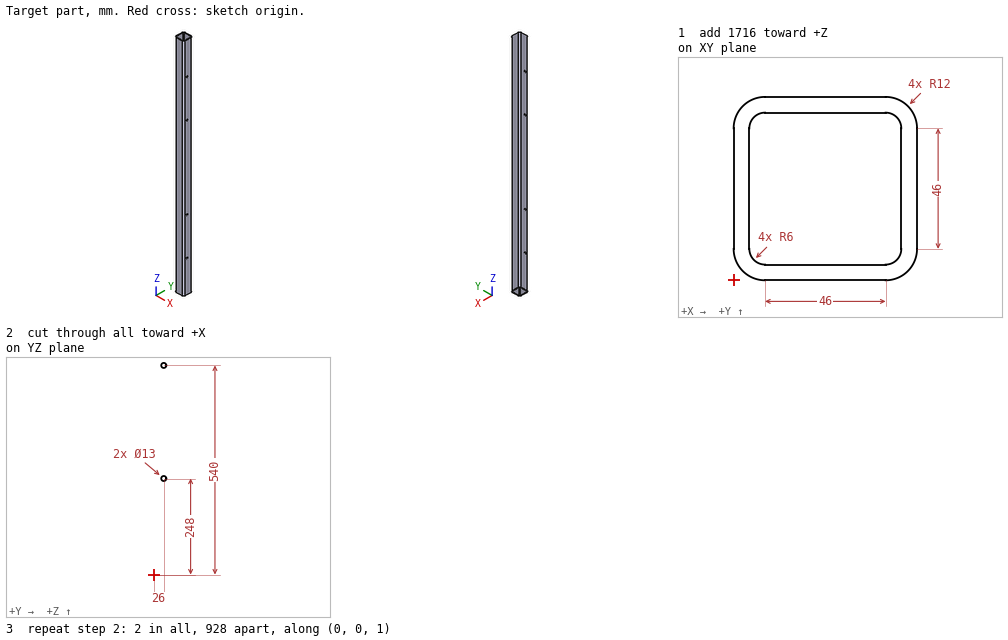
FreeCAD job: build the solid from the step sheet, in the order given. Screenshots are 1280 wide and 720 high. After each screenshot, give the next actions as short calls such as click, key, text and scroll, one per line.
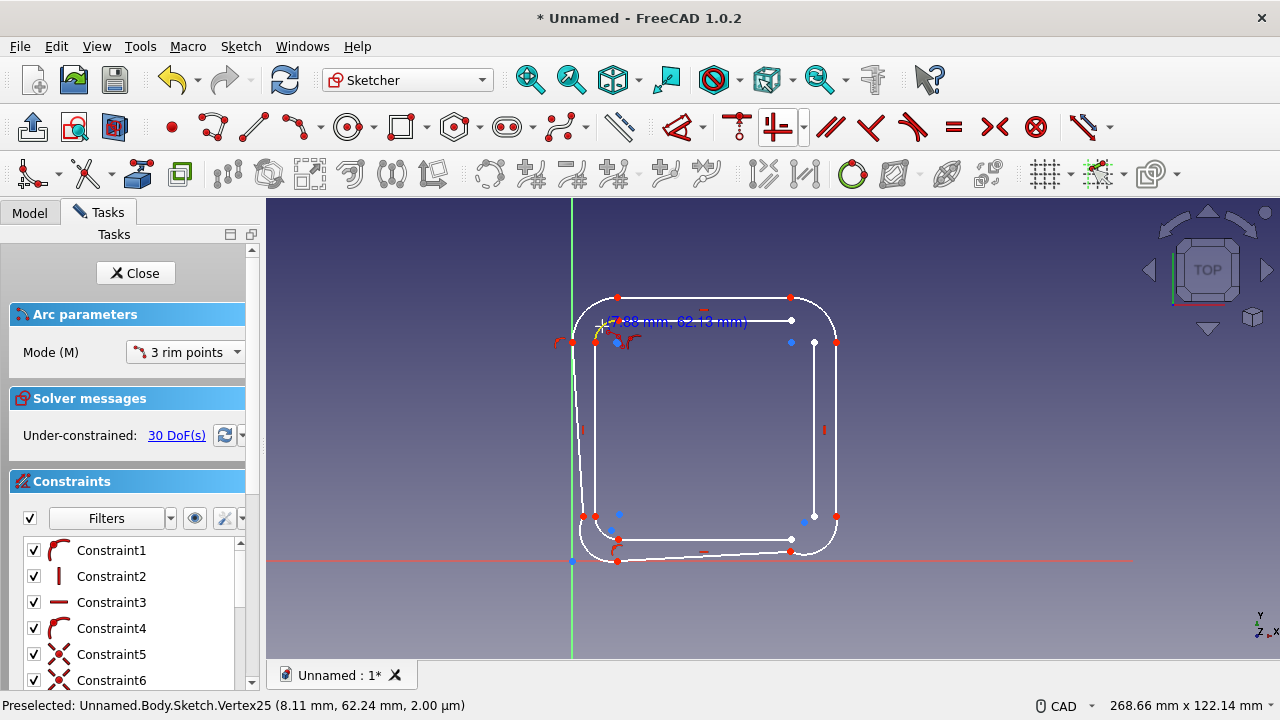
click(791, 321)
click(814, 343)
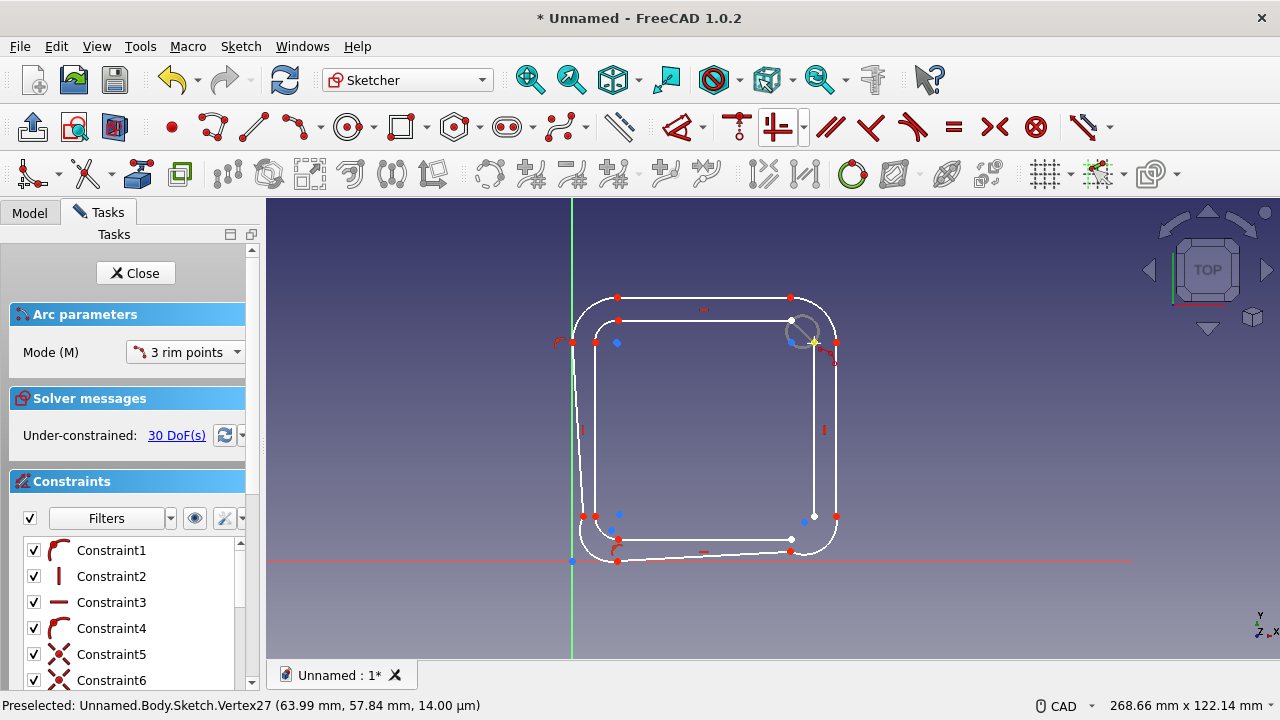
scroll(807, 326, up, 5)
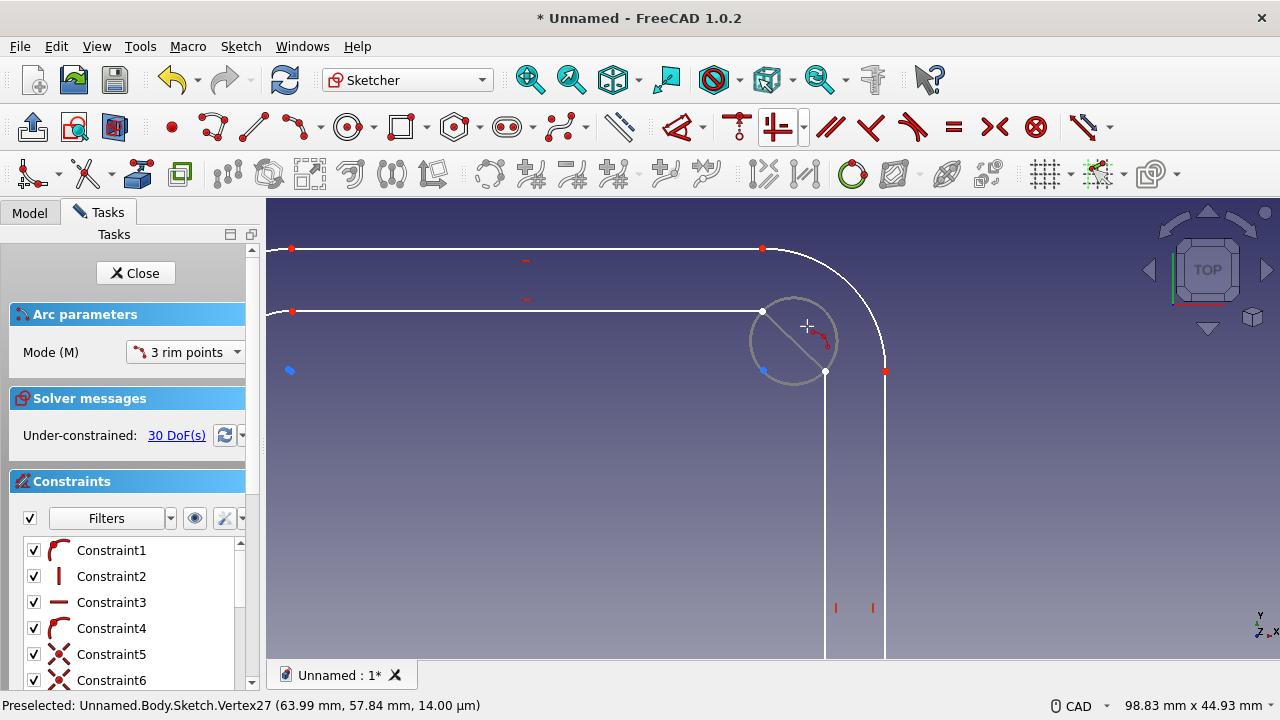
click(807, 326)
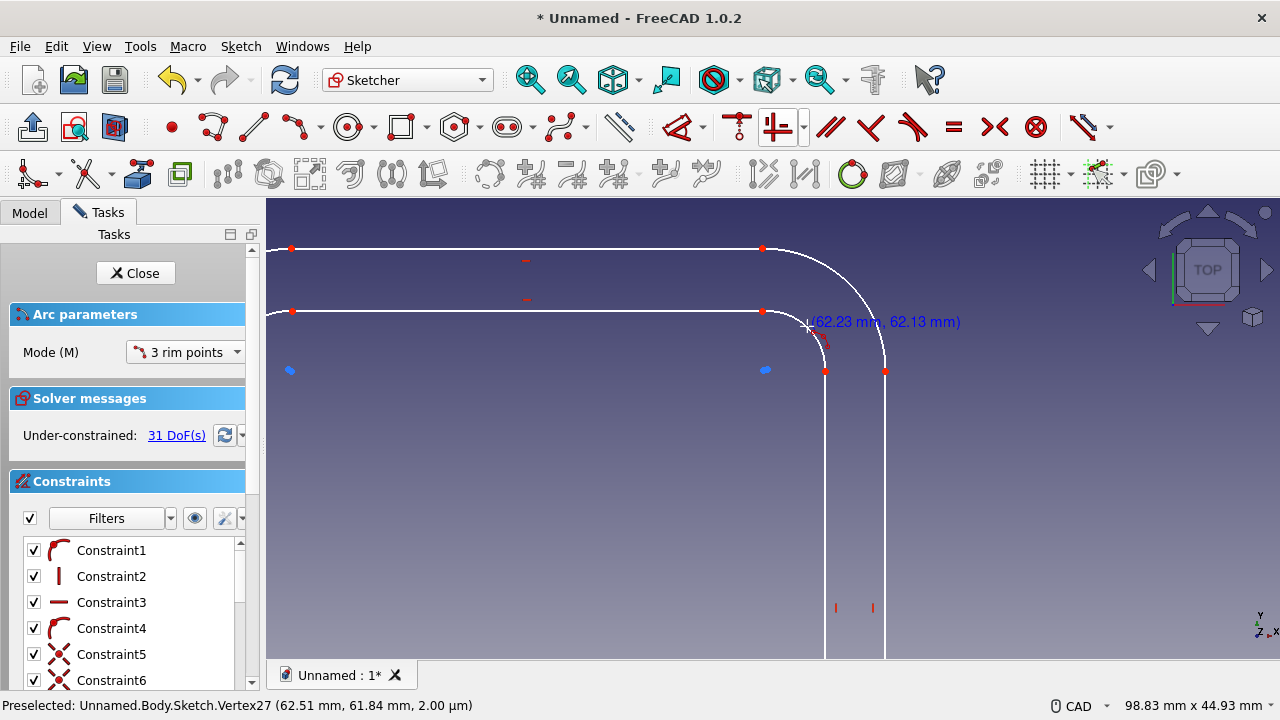
scroll(807, 326, down, 5)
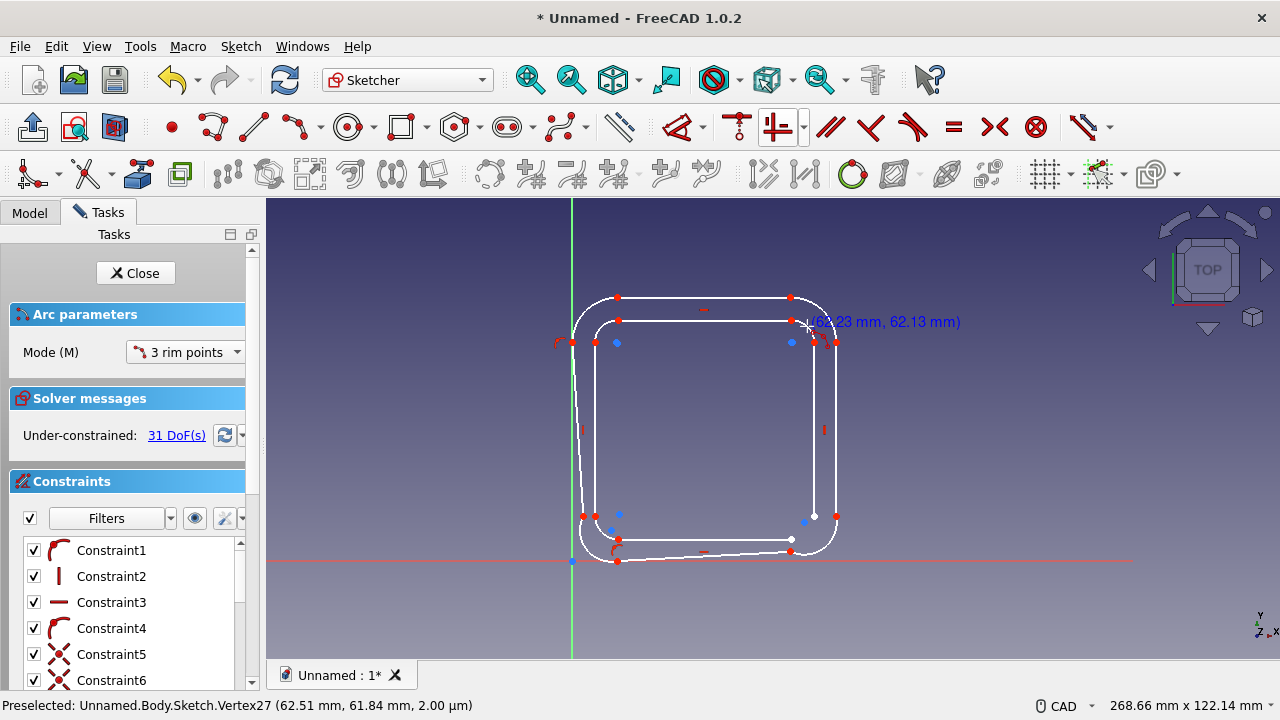
click(814, 517)
click(791, 540)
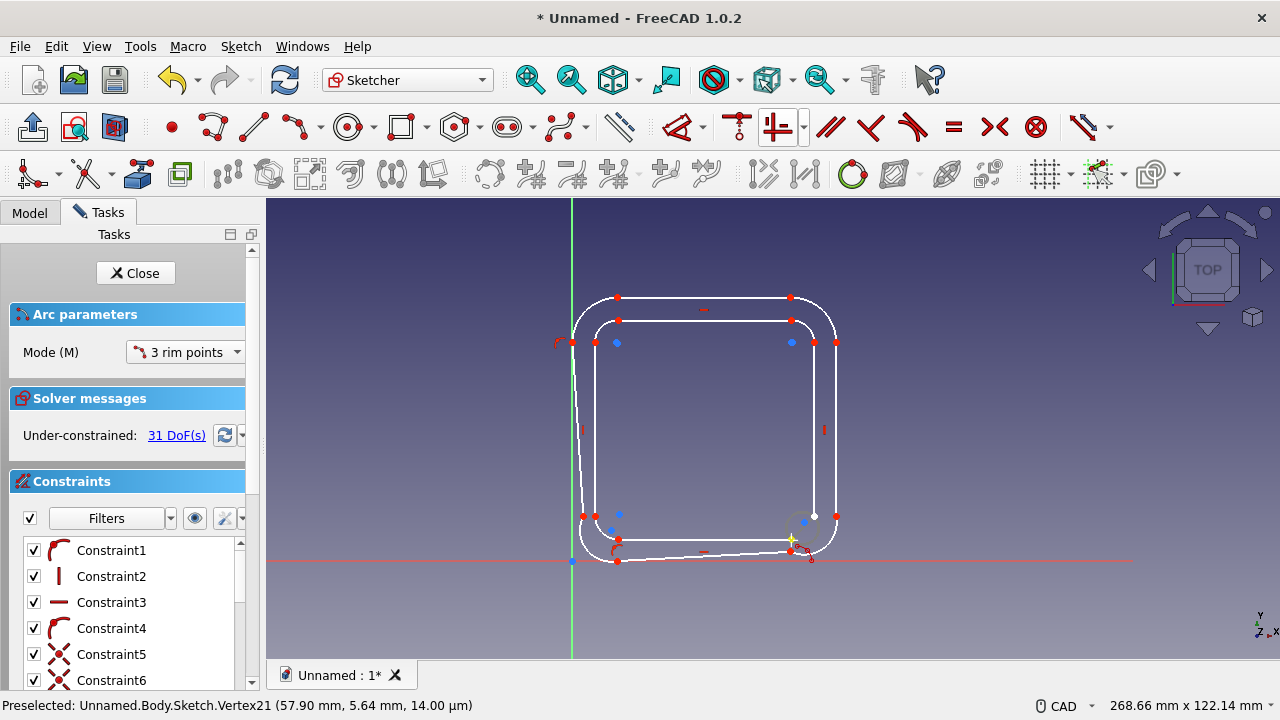
scroll(807, 532, up, 5)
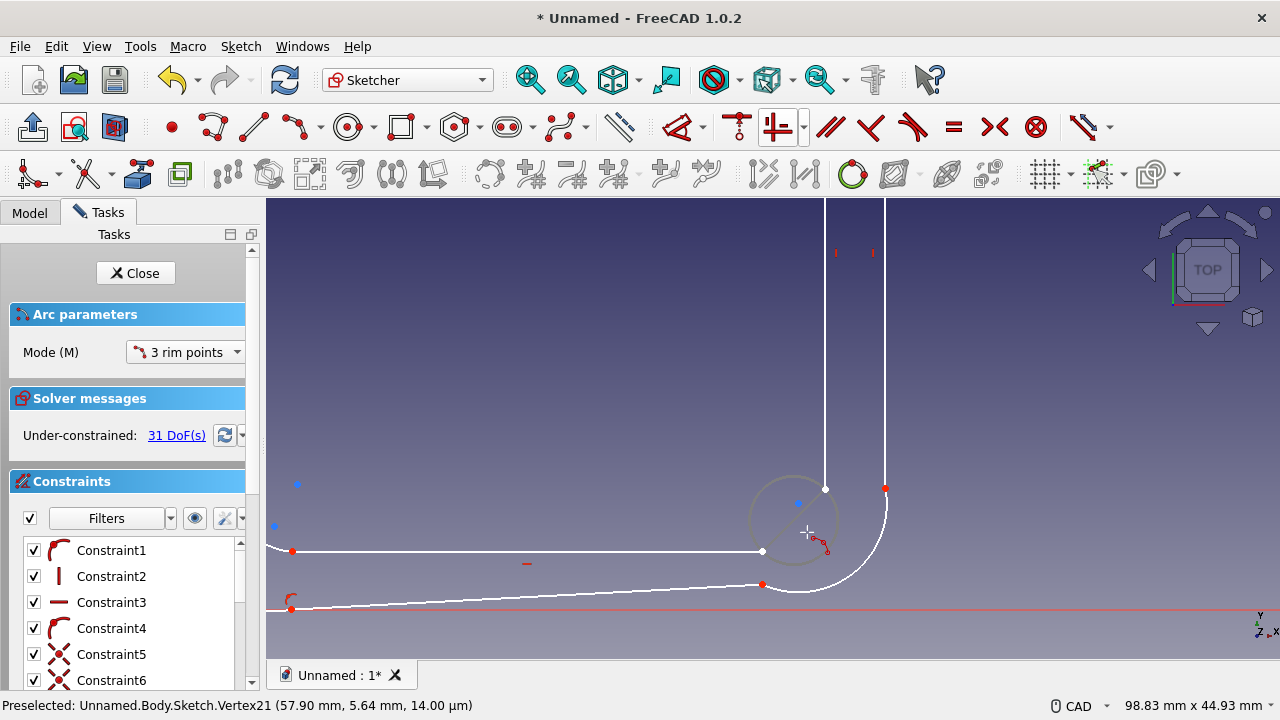
click(807, 530)
key(Escape)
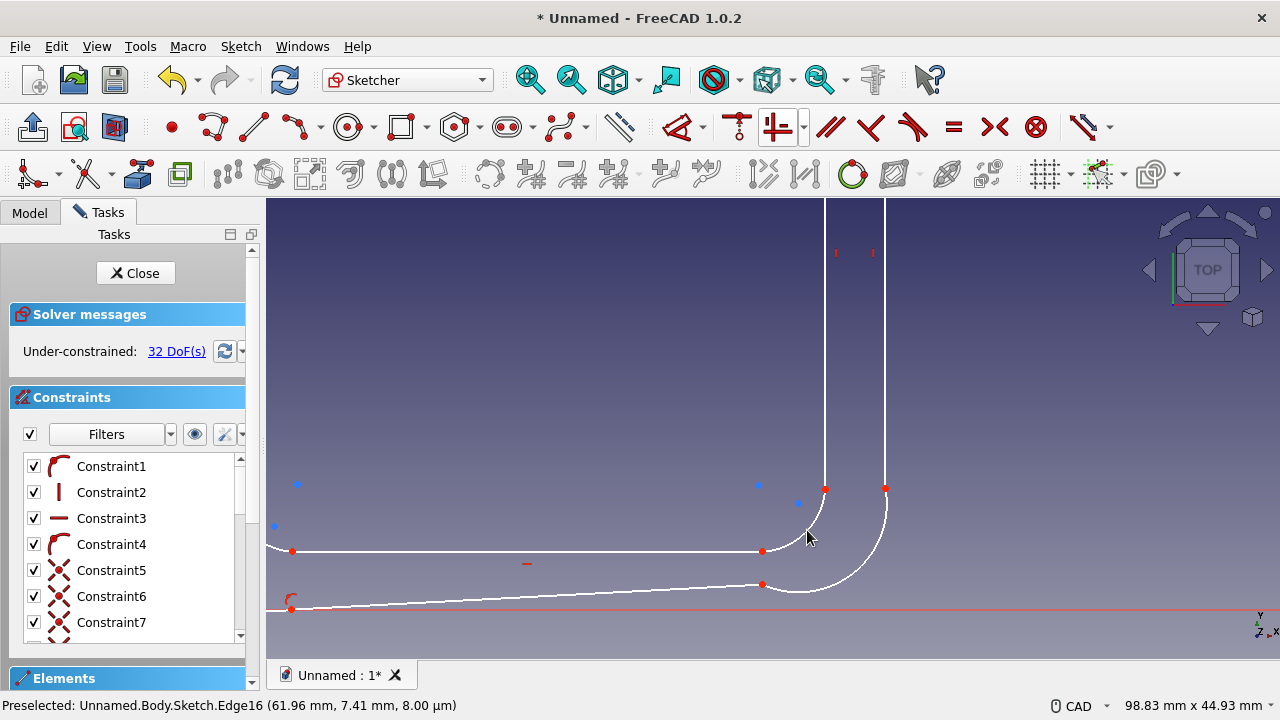
click(621, 592)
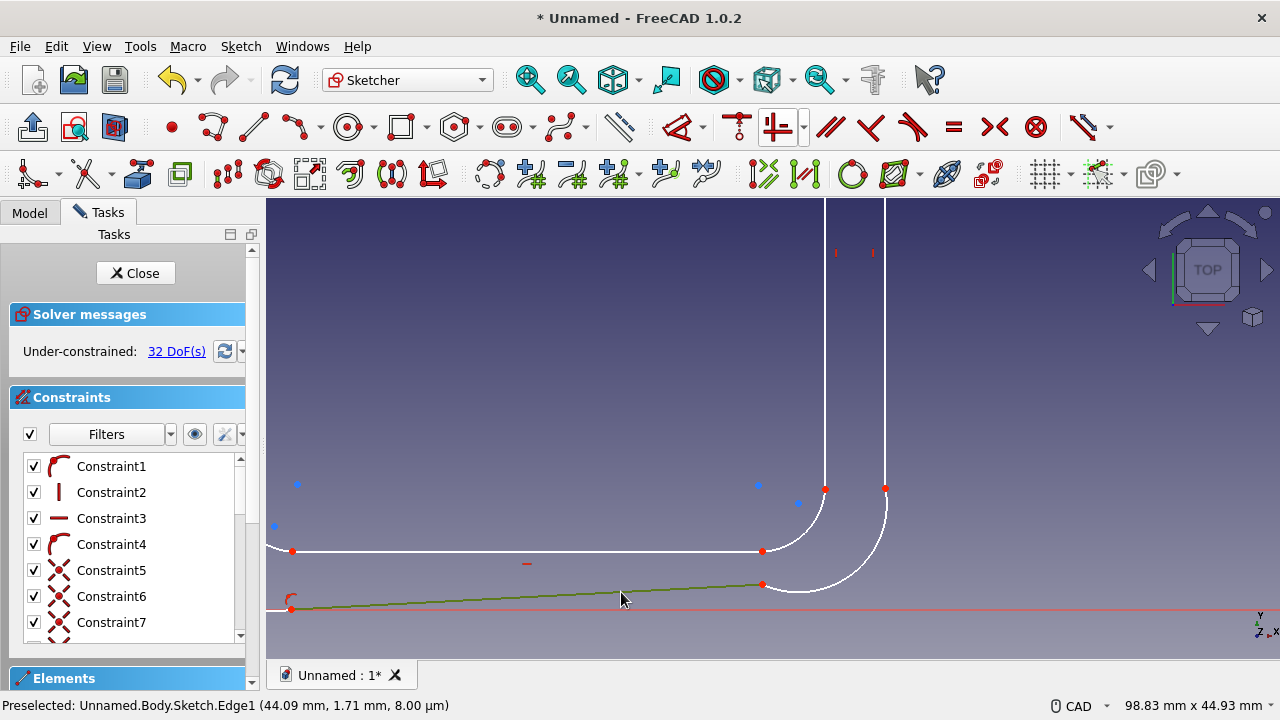
click(819, 590)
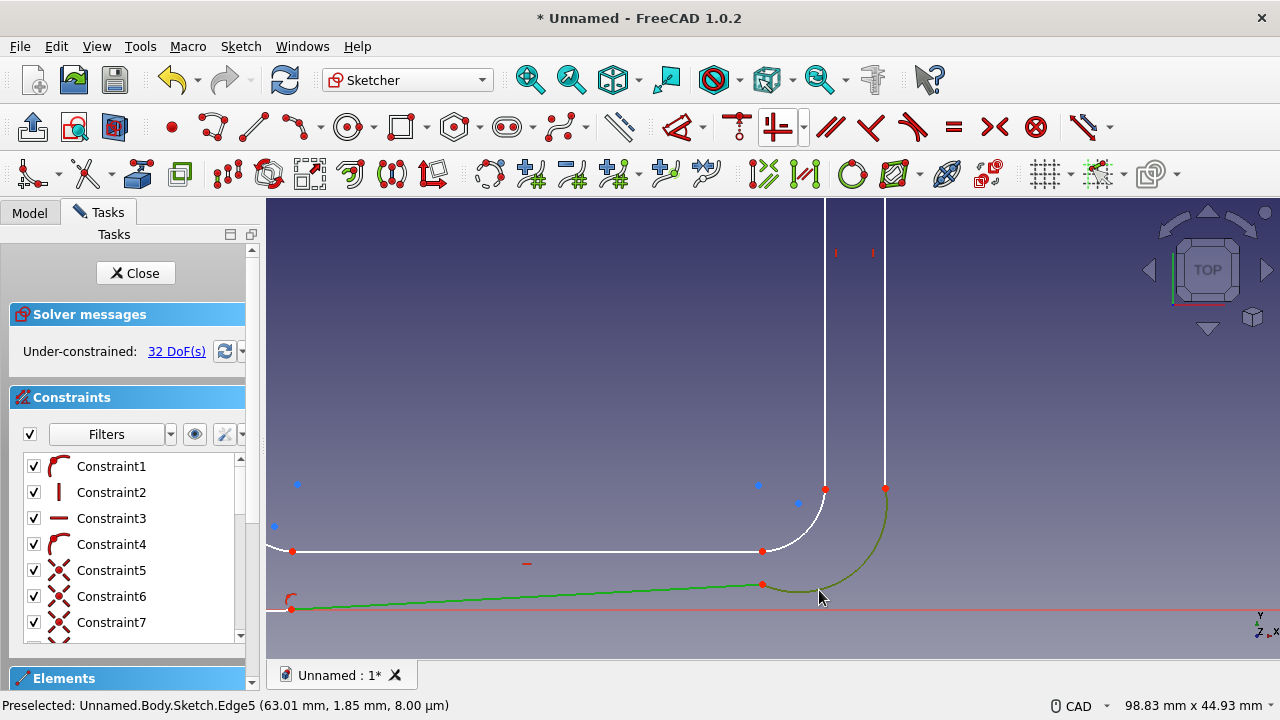
click(913, 128)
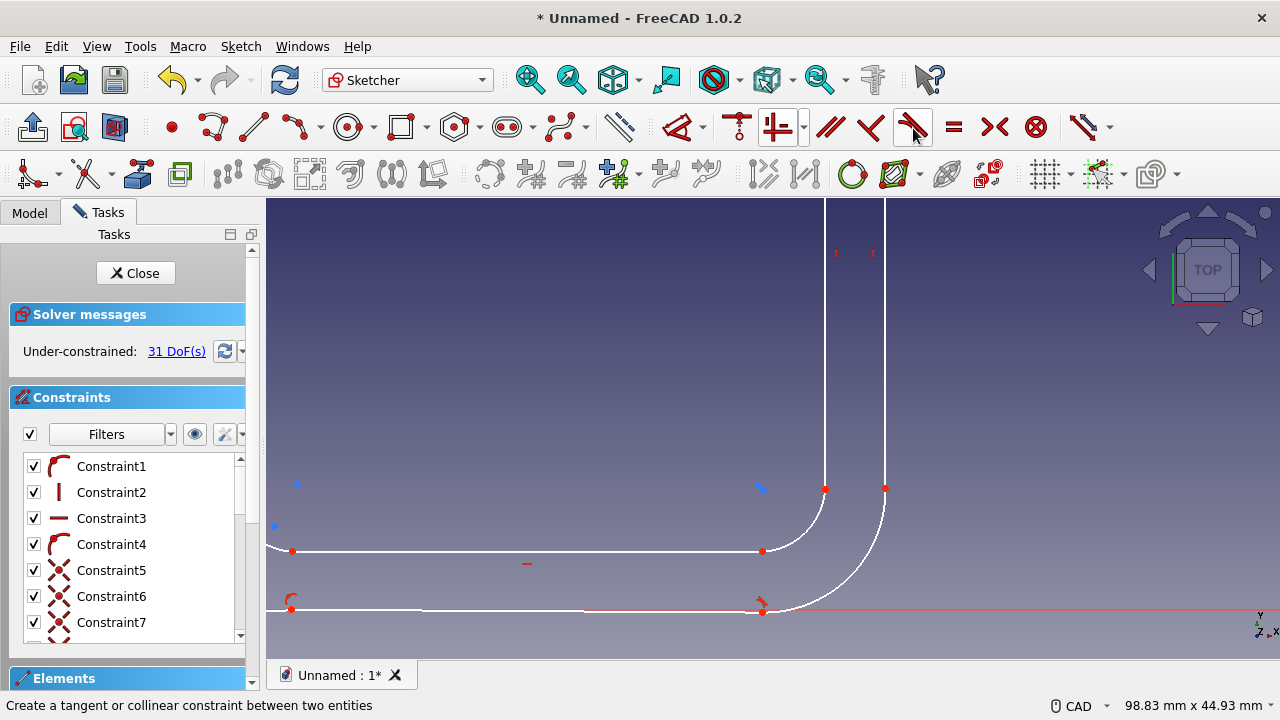
click(433, 611)